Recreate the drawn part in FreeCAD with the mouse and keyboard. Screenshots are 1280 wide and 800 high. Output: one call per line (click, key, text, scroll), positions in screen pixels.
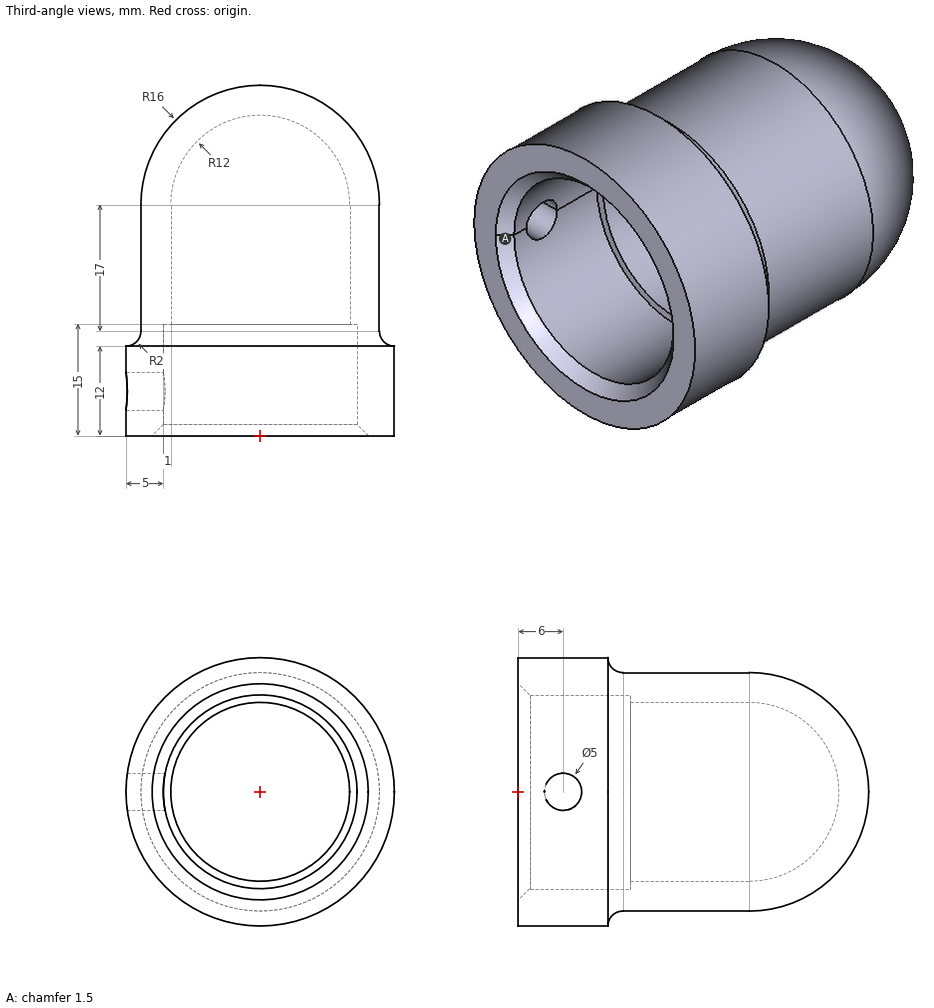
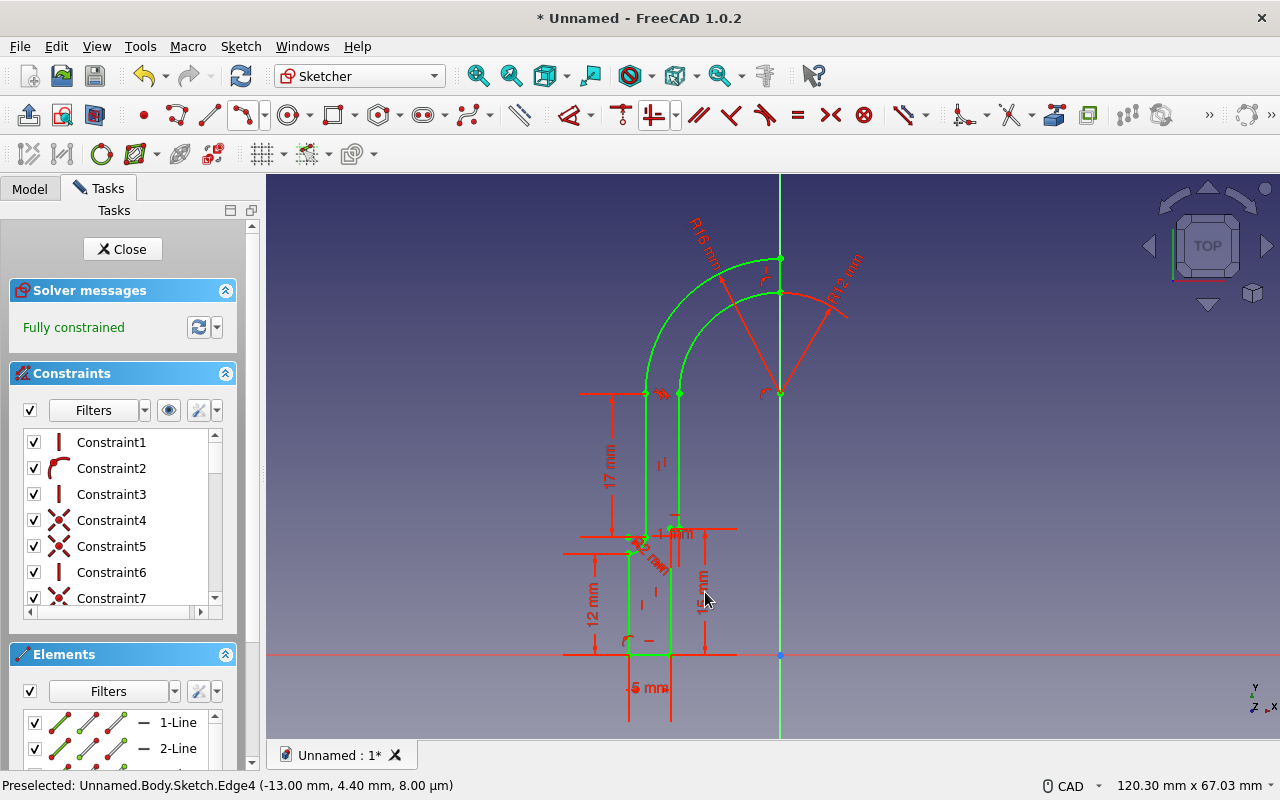
click(123, 249)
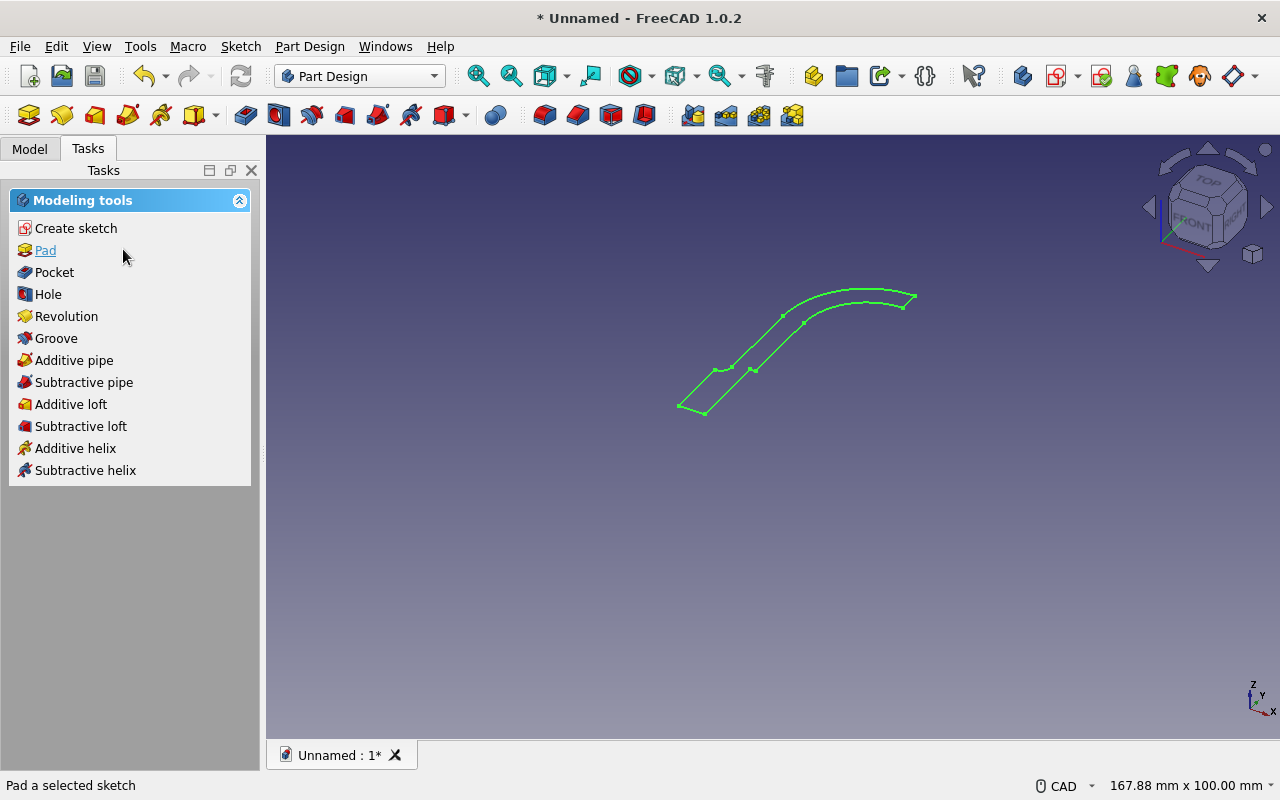
click(62, 116)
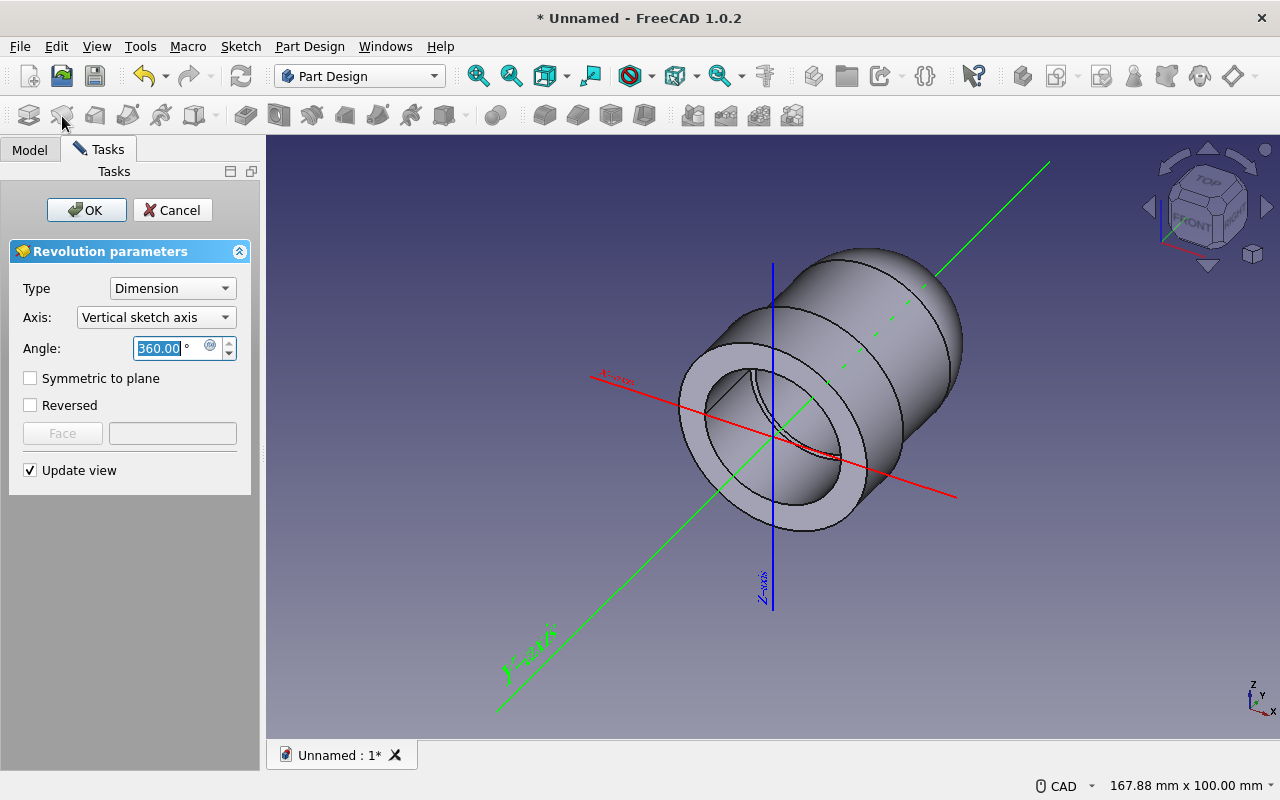
click(87, 210)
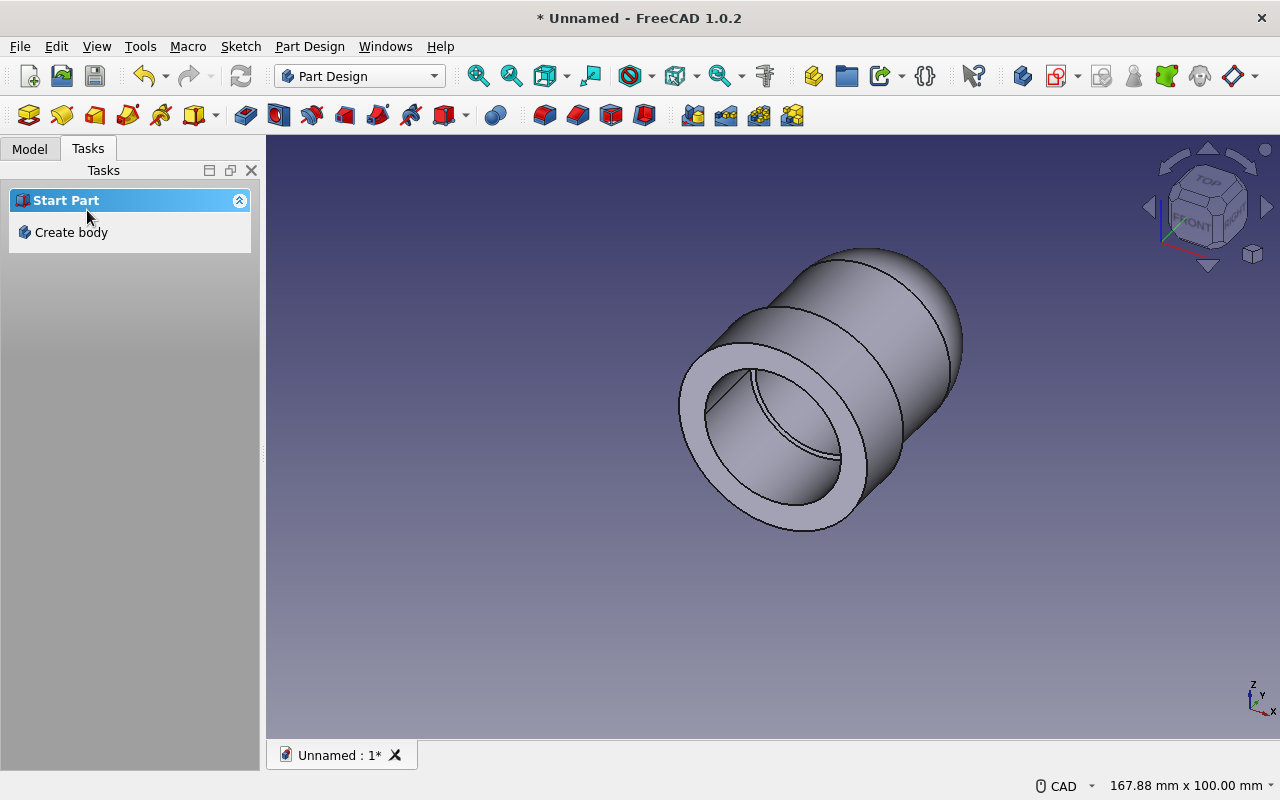
click(1056, 76)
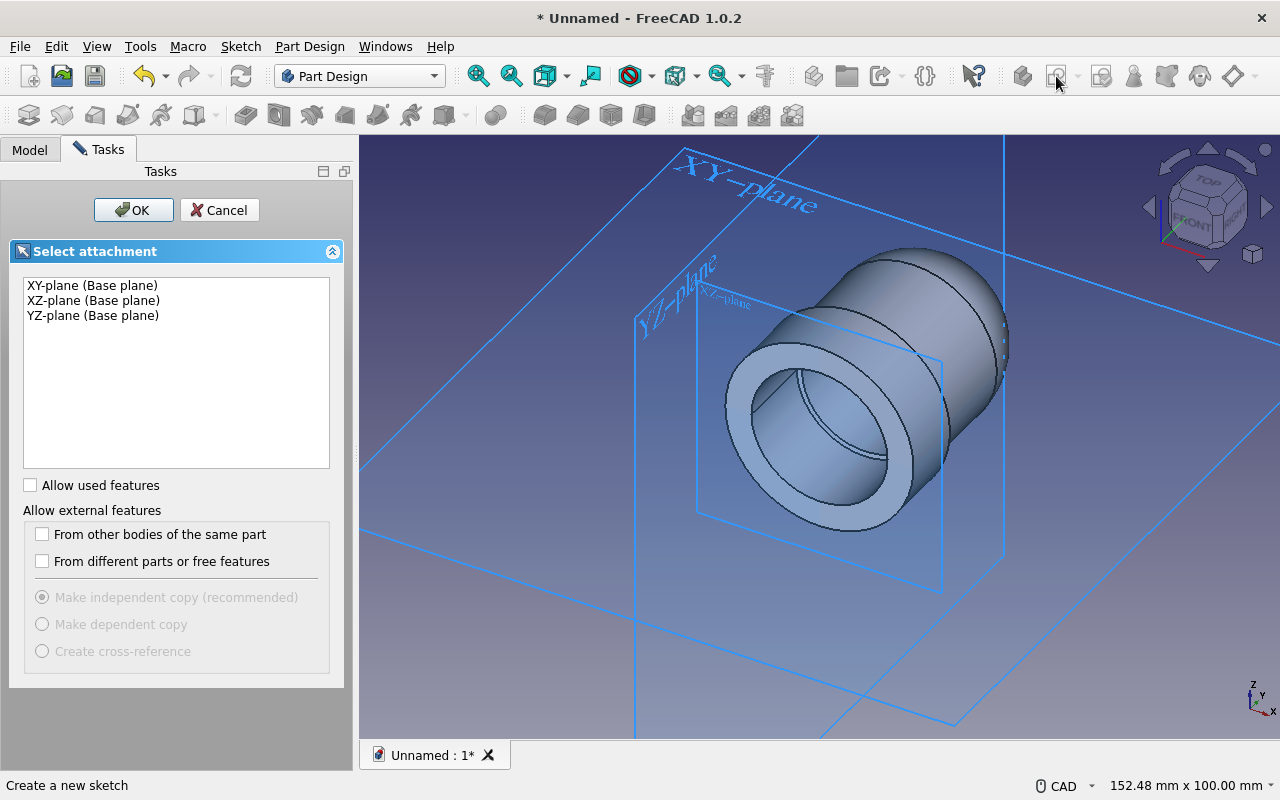
click(84, 316)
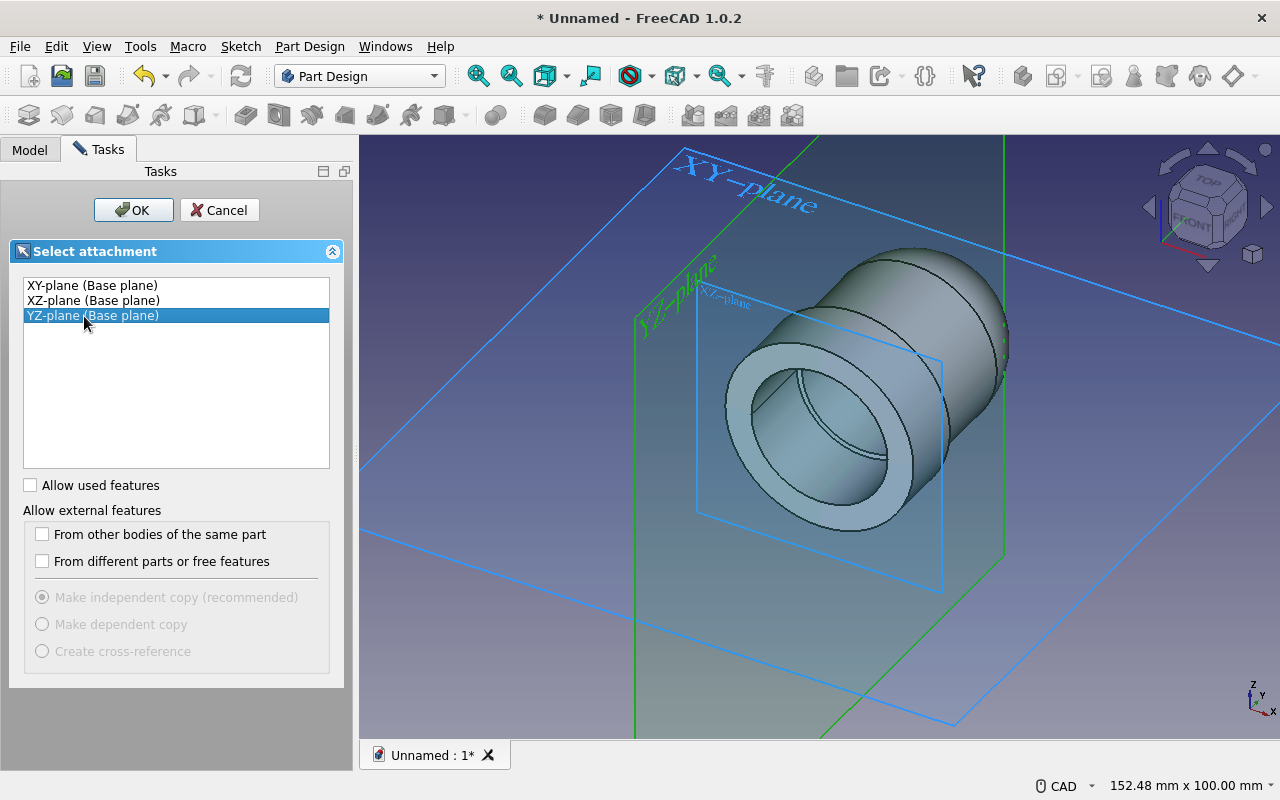
click(134, 210)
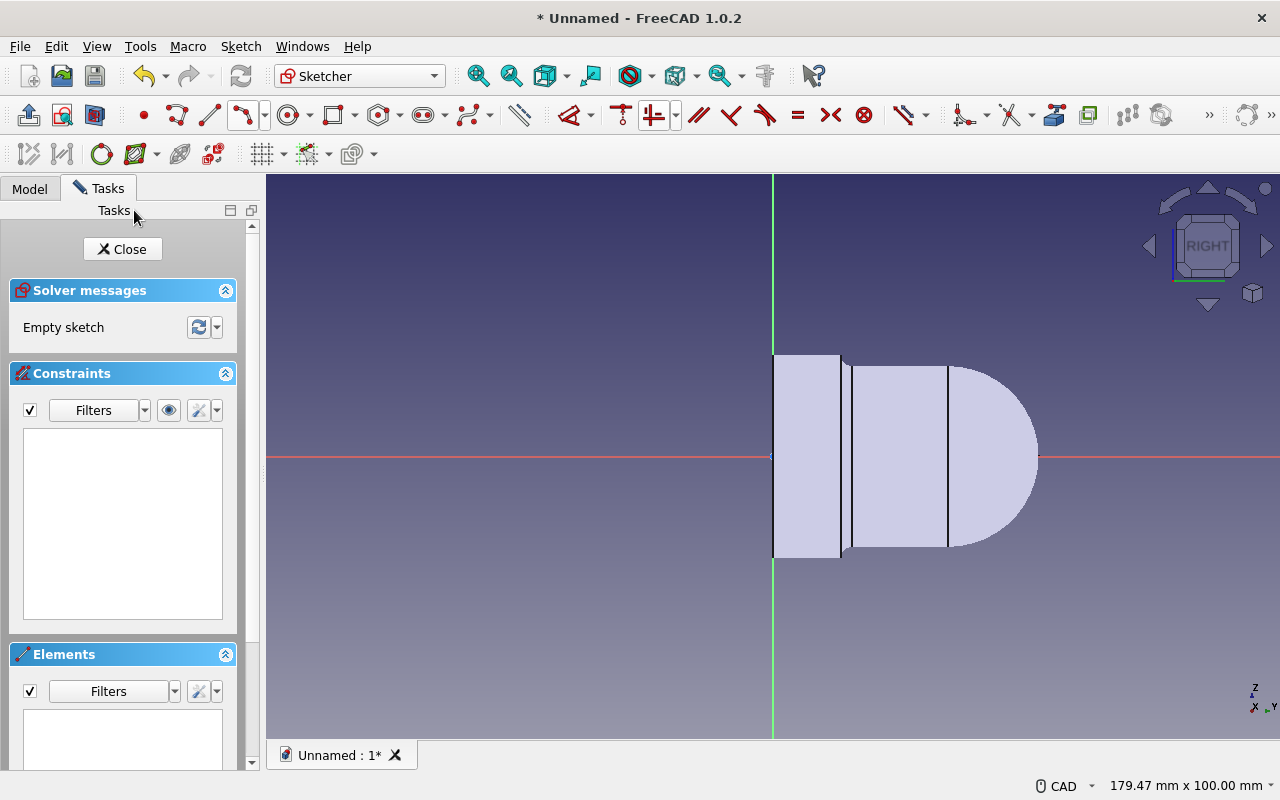
click(95, 116)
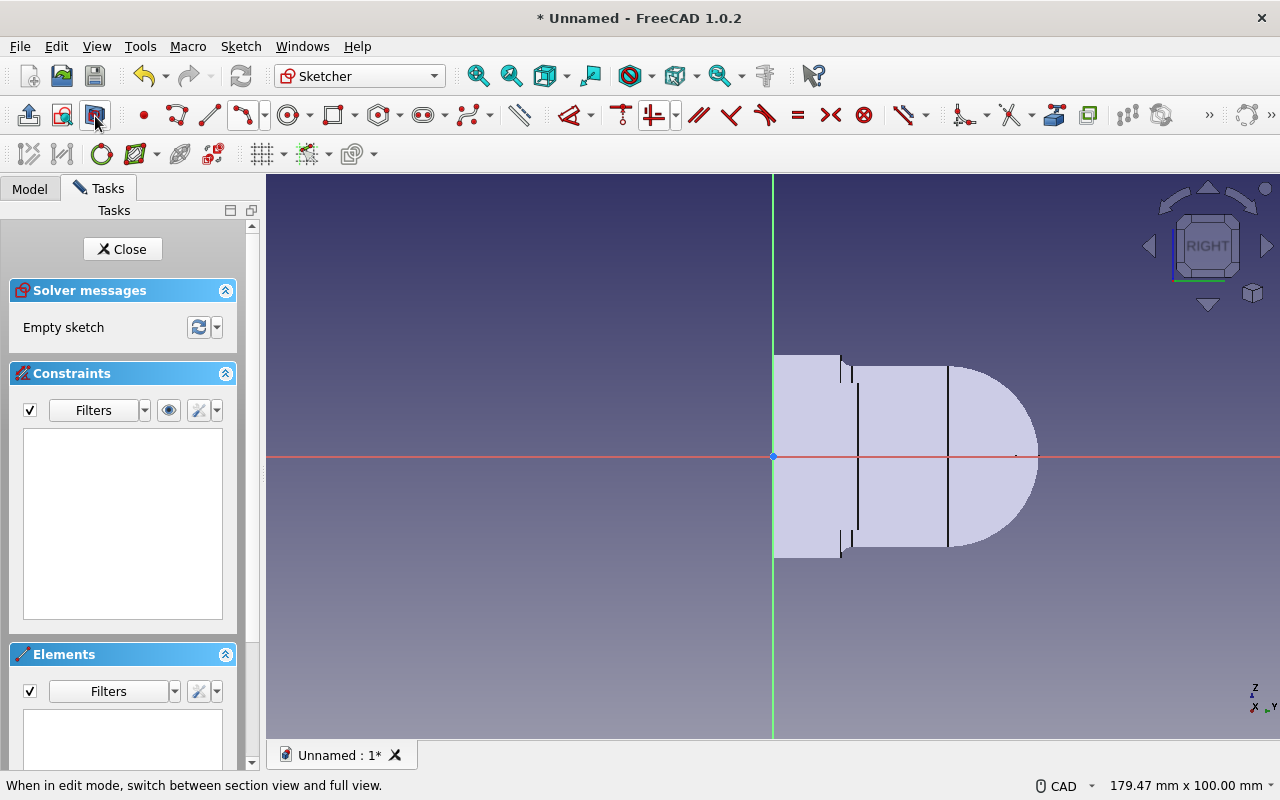
scroll(806, 456, up, 12)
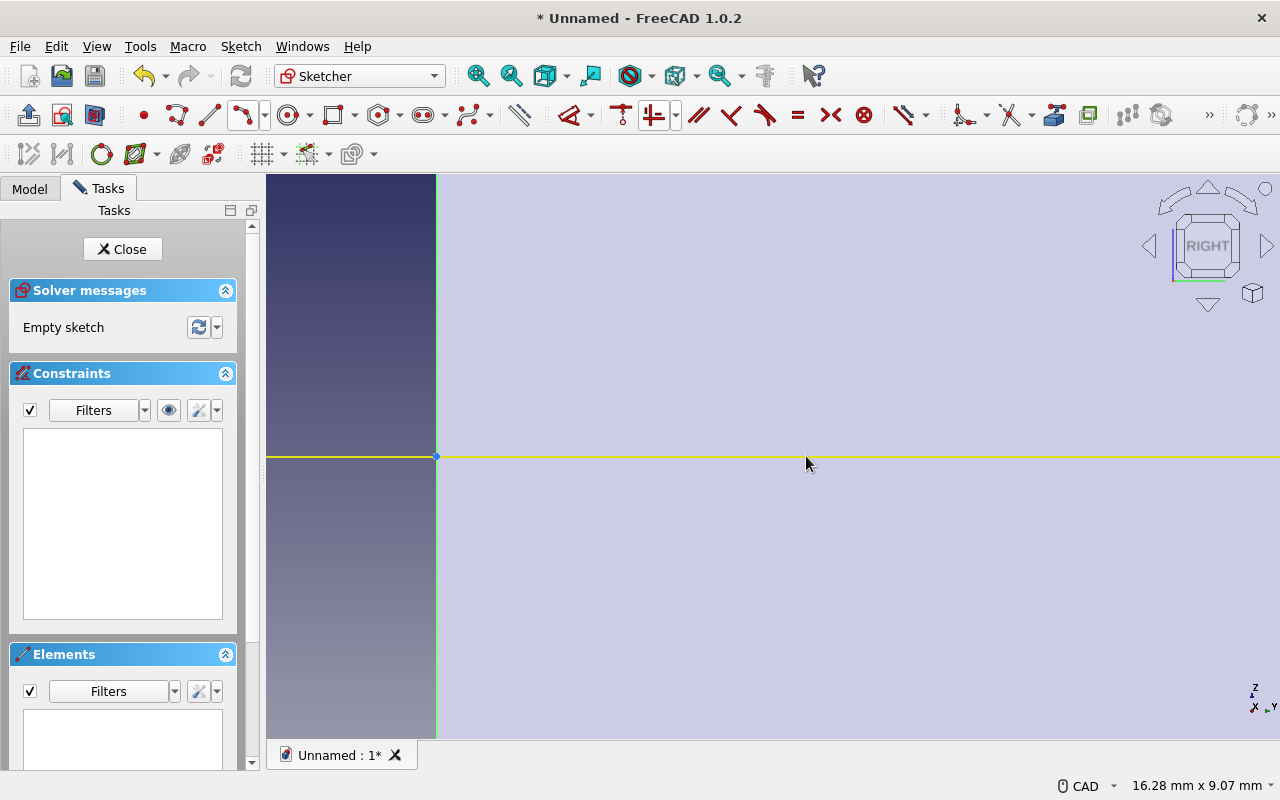
click(288, 116)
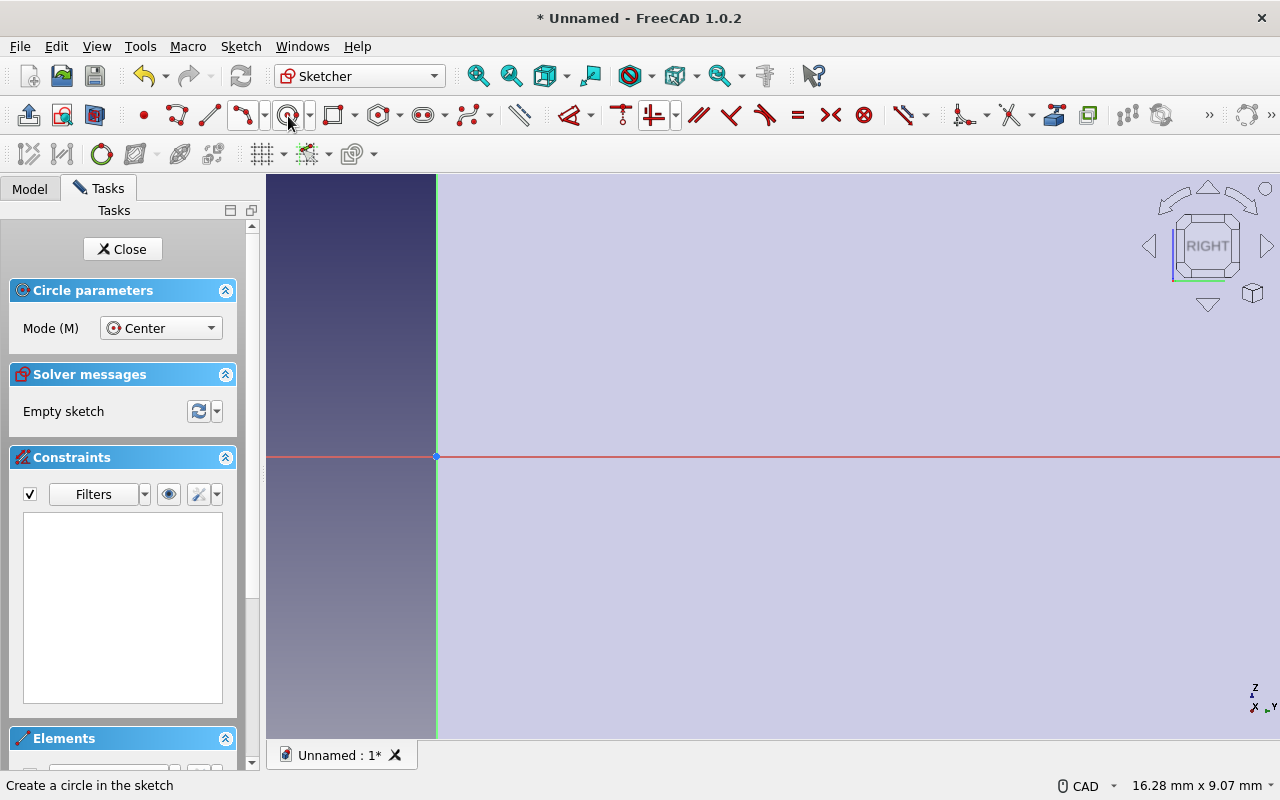
click(811, 456)
move(921, 346)